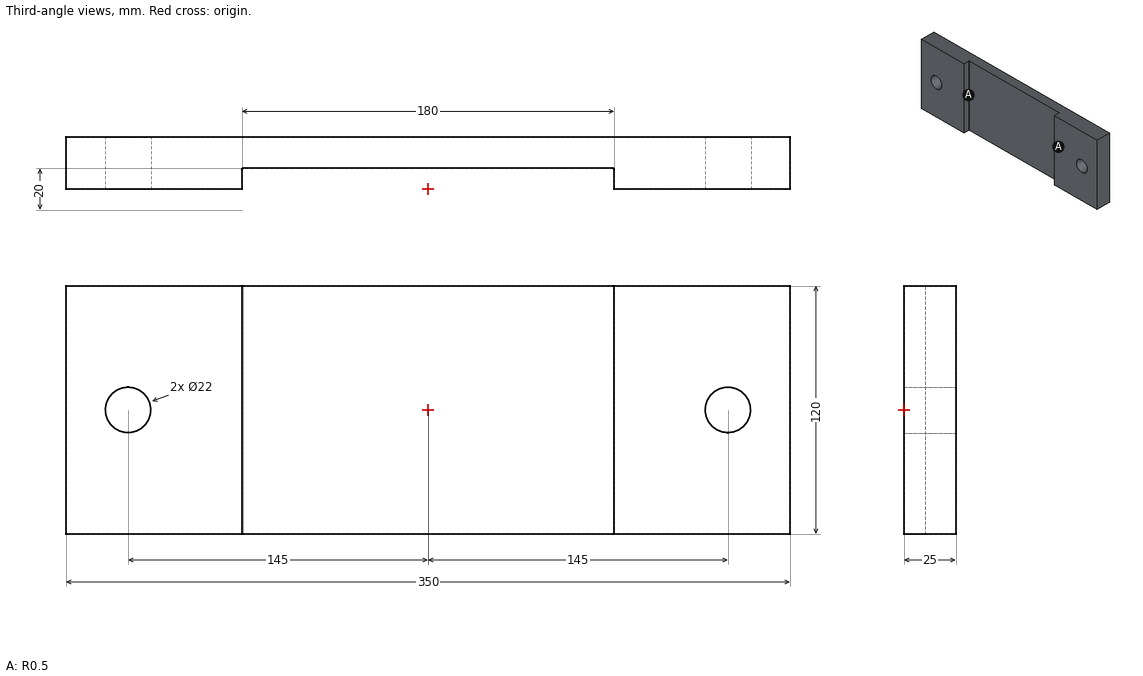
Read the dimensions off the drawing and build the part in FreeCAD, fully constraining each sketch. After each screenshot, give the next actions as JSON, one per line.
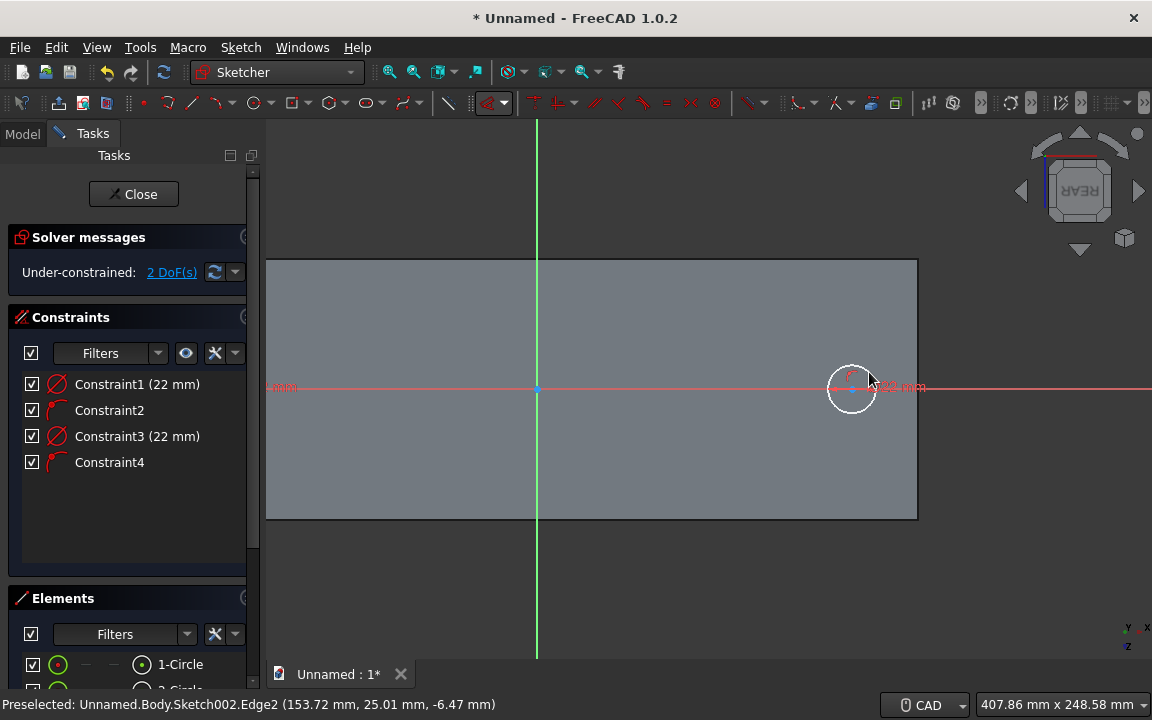
{"action": "left_click", "coordinate": [488, 104]}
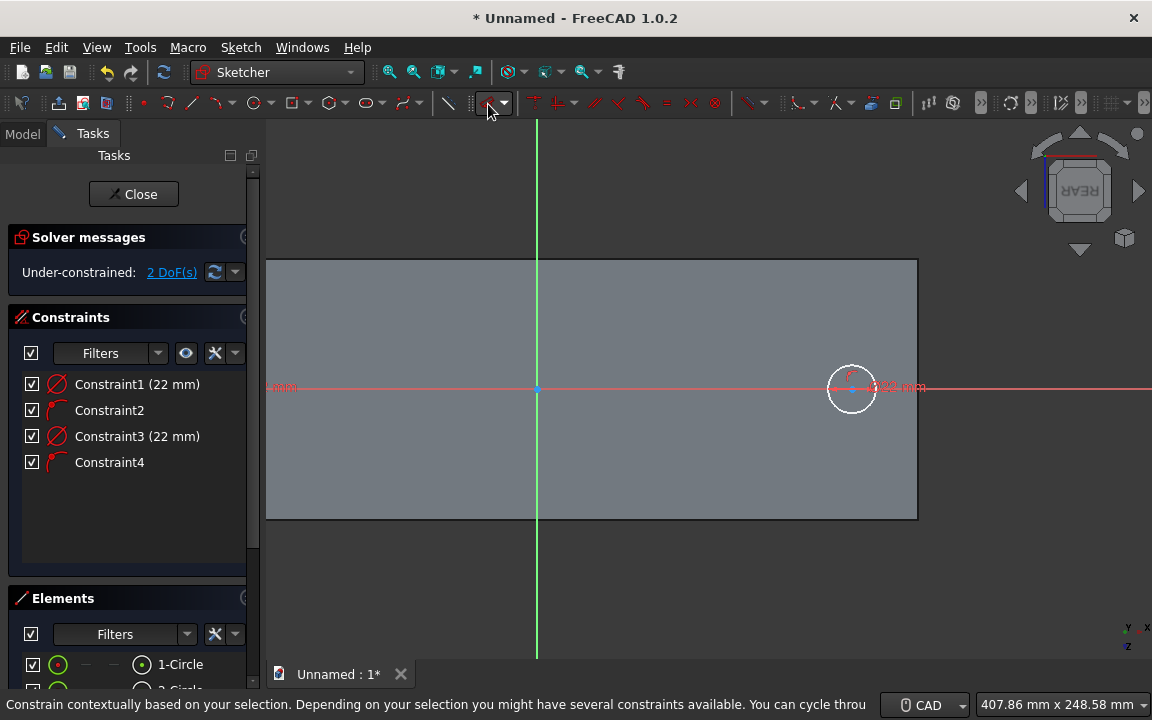
{"action": "scroll", "coordinate": [850, 388], "scroll_direction": "down", "scroll_amount": 2}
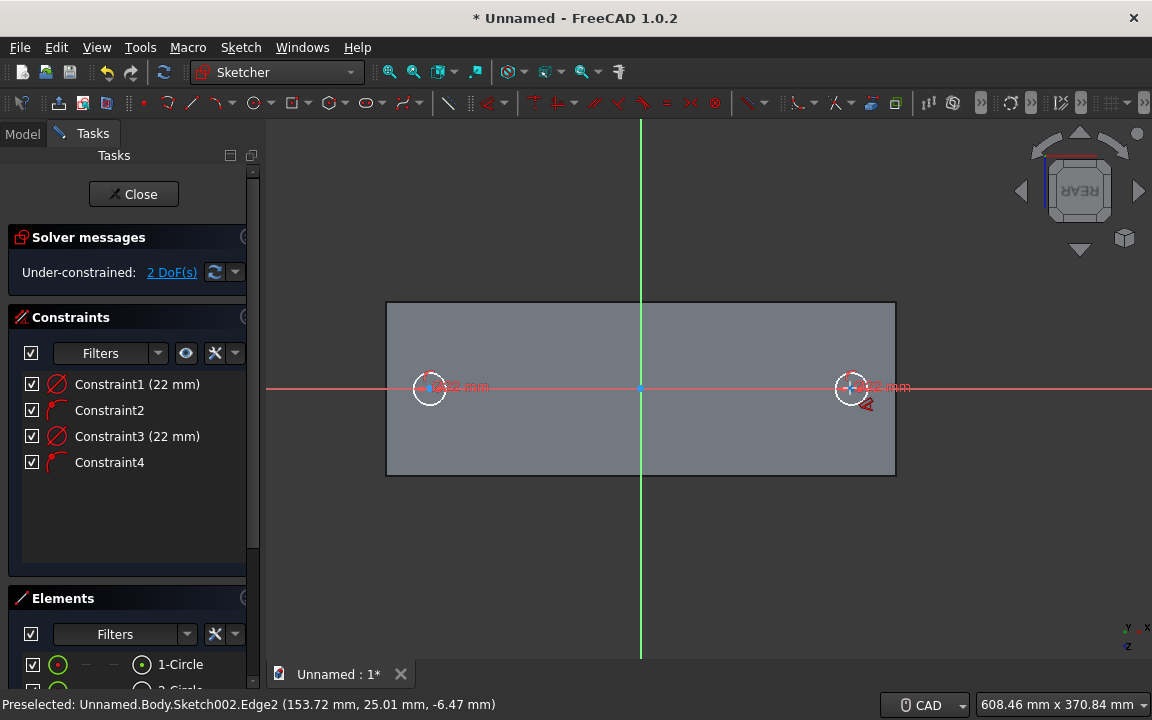
{"action": "left_click", "coordinate": [430, 389]}
{"action": "left_click", "coordinate": [535, 423]}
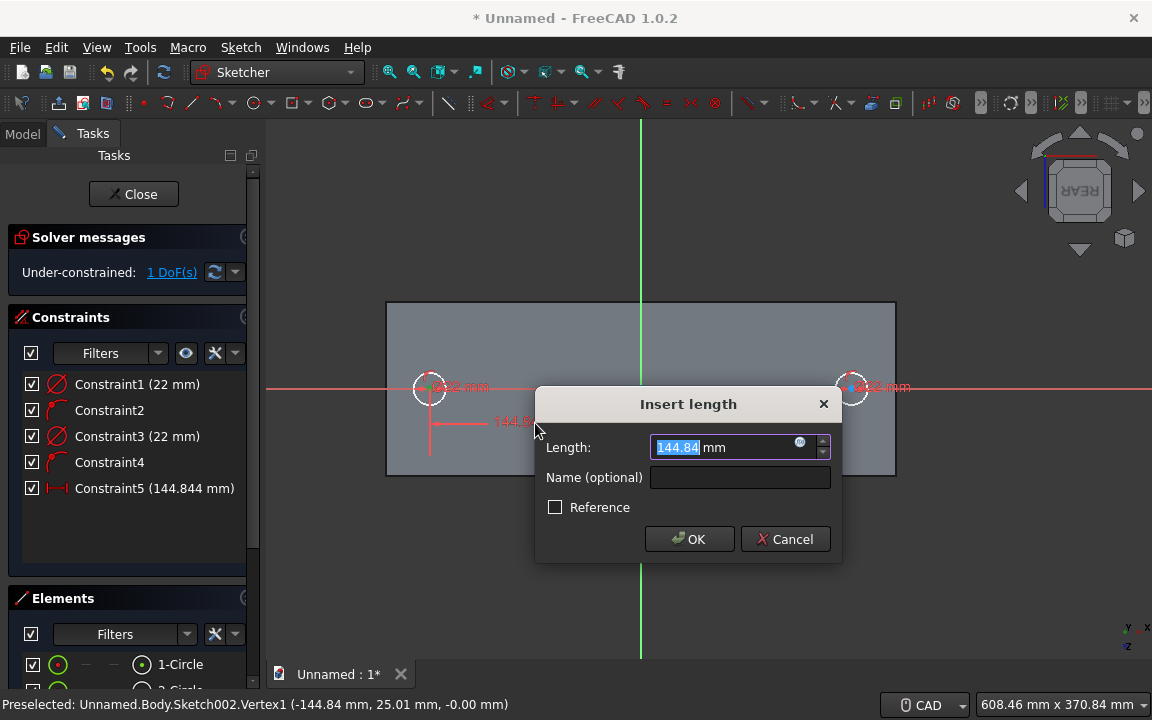
{"action": "type", "text": "145"}
{"action": "key", "text": "Return"}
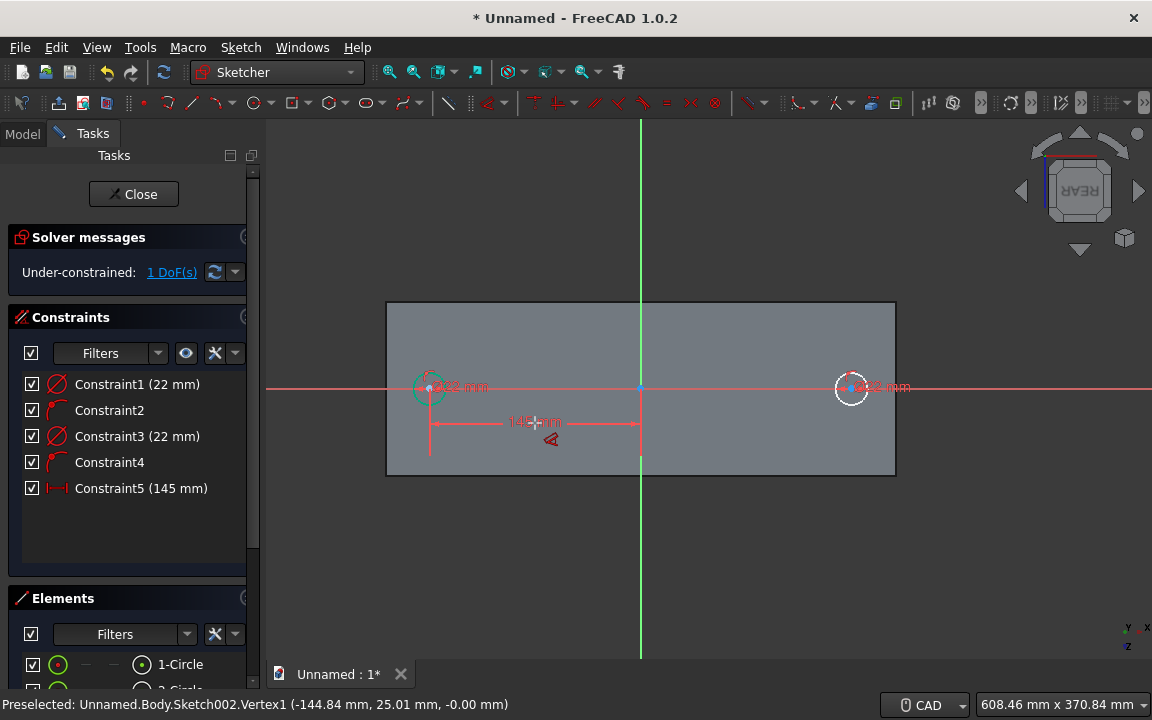
{"action": "left_click", "coordinate": [852, 389]}
{"action": "left_click", "coordinate": [746, 423]}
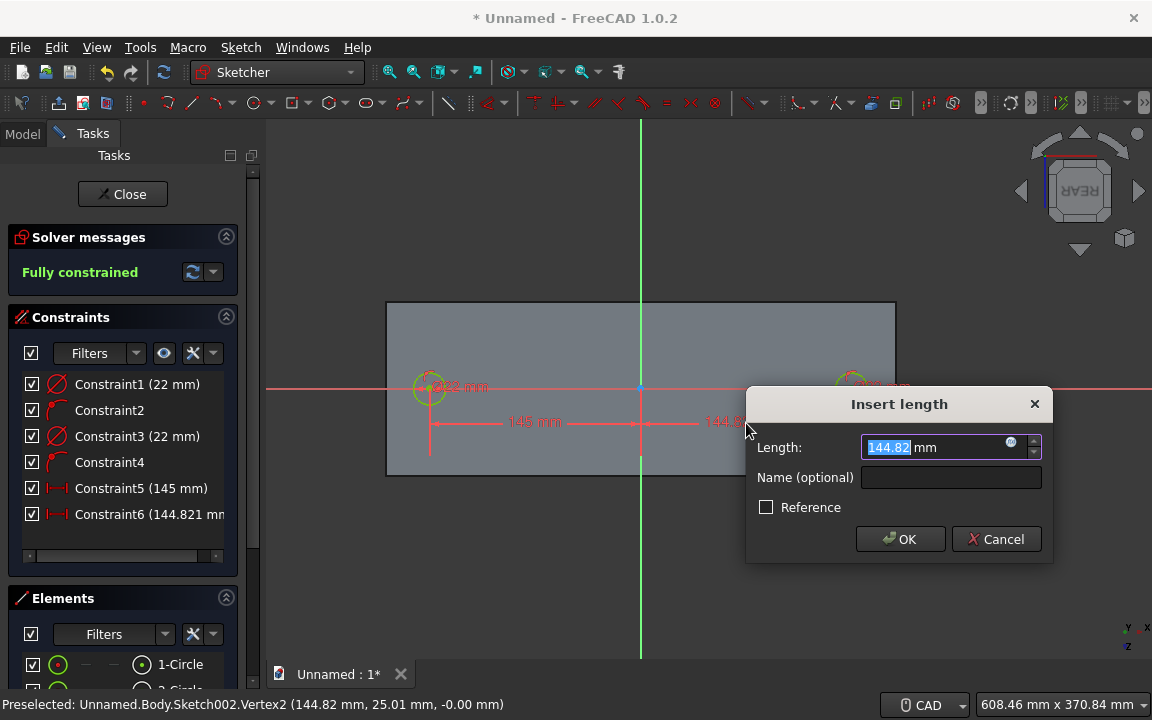
{"action": "type", "text": "145"}
{"action": "key", "text": "Return"}
{"action": "key", "text": "Escape"}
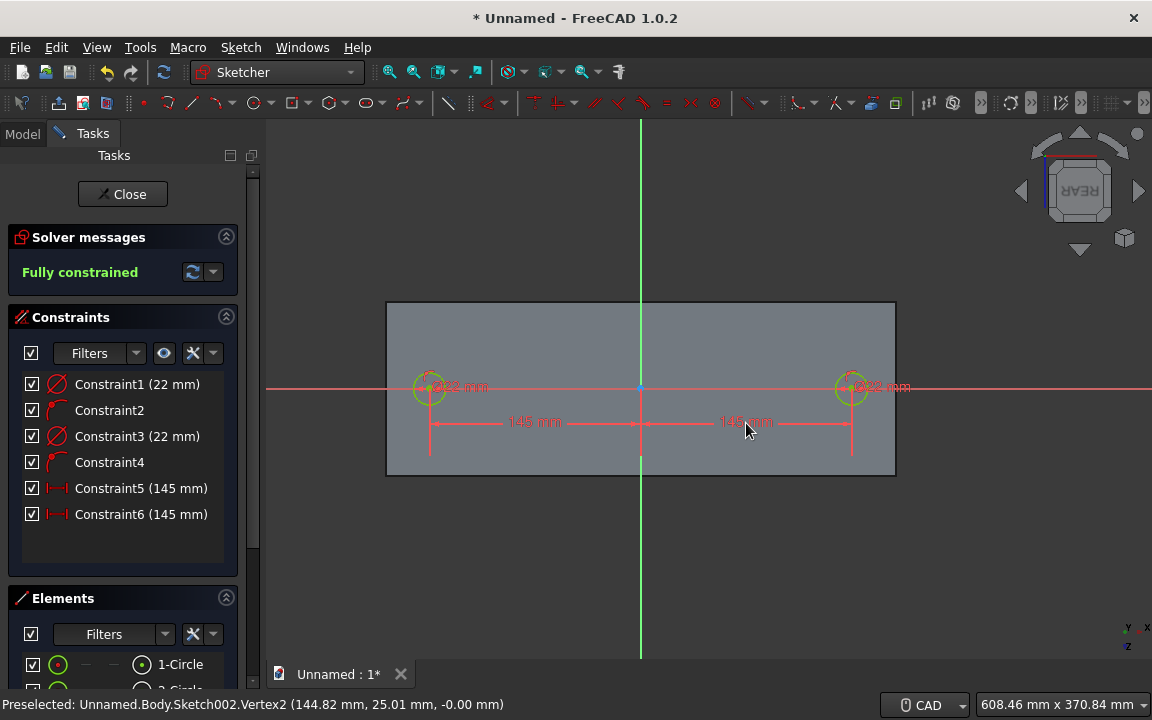
{"action": "left_click", "coordinate": [123, 194]}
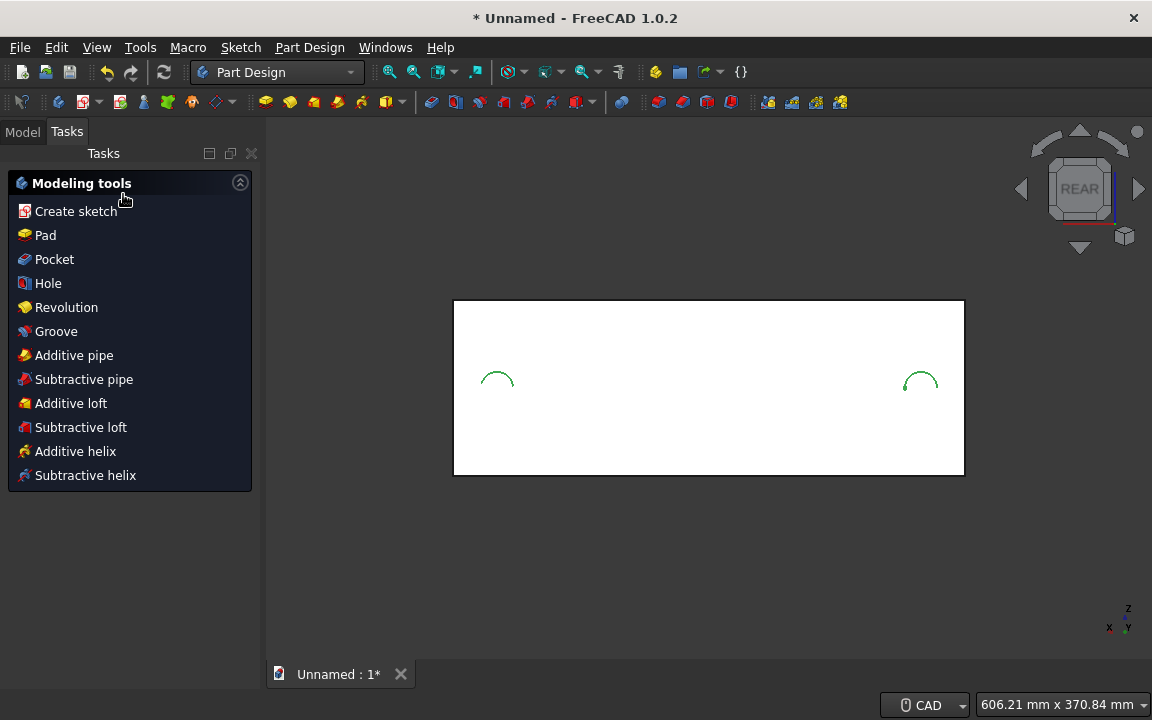
{"action": "left_click", "coordinate": [432, 102]}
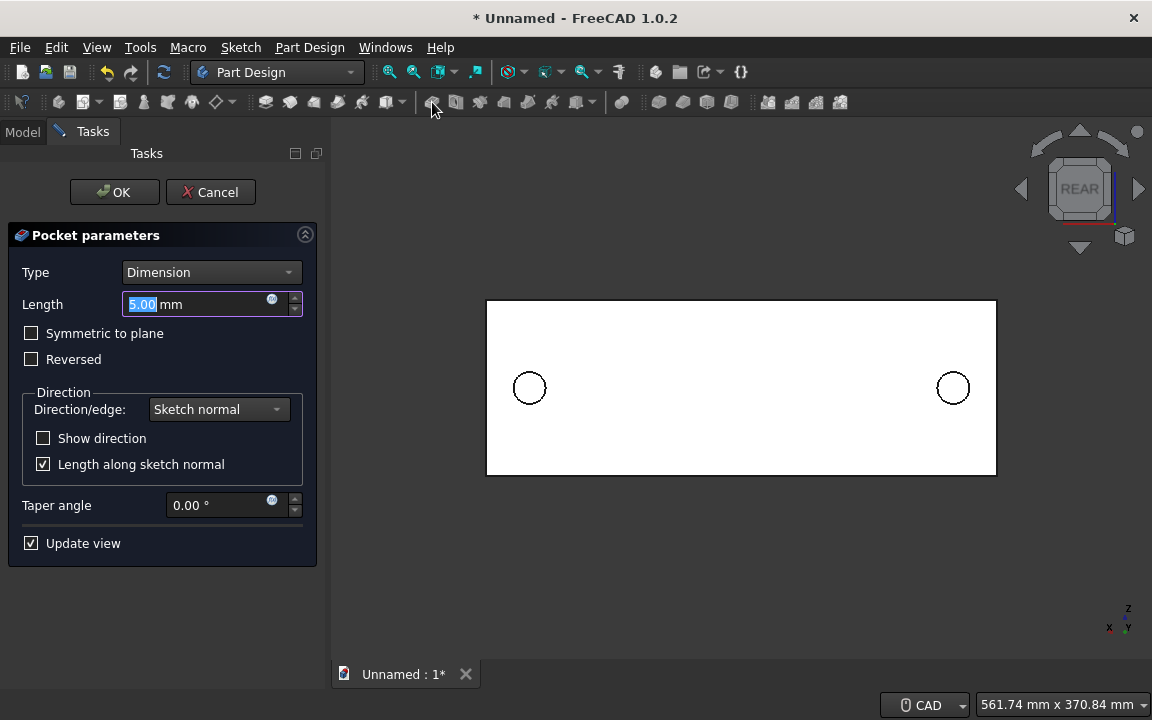
{"action": "type", "text": "25"}
{"action": "key", "text": "Tab"}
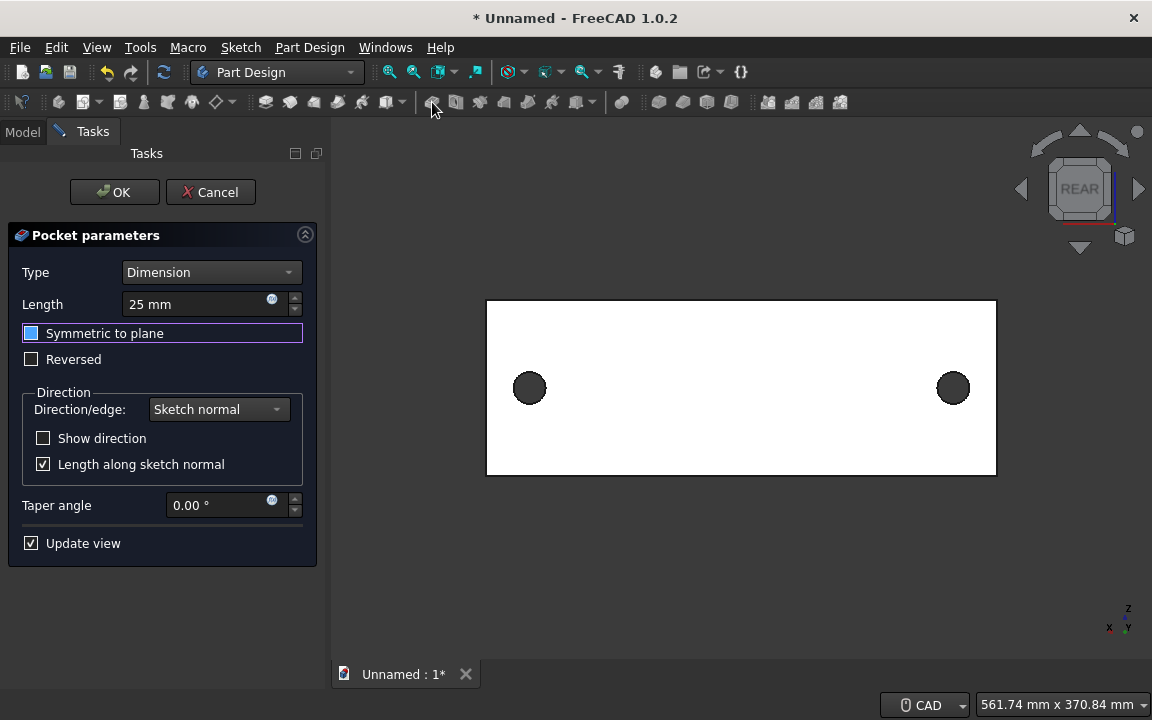
{"action": "left_click", "coordinate": [115, 192]}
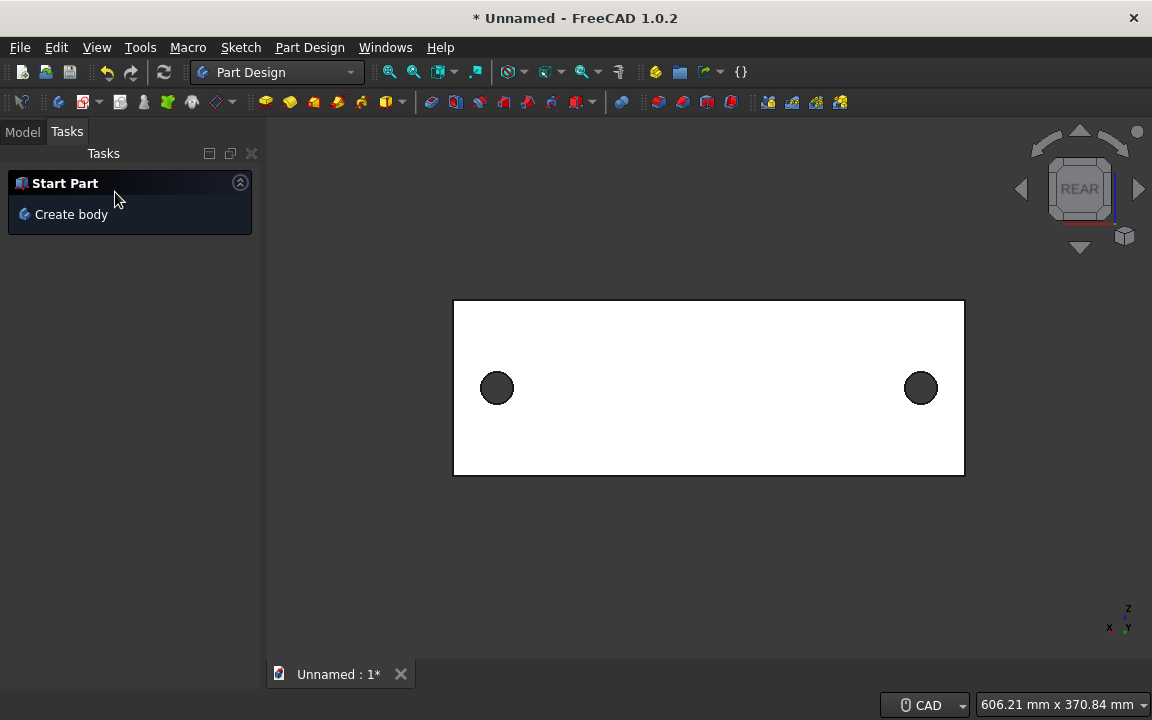
{"action": "key", "text": "0"}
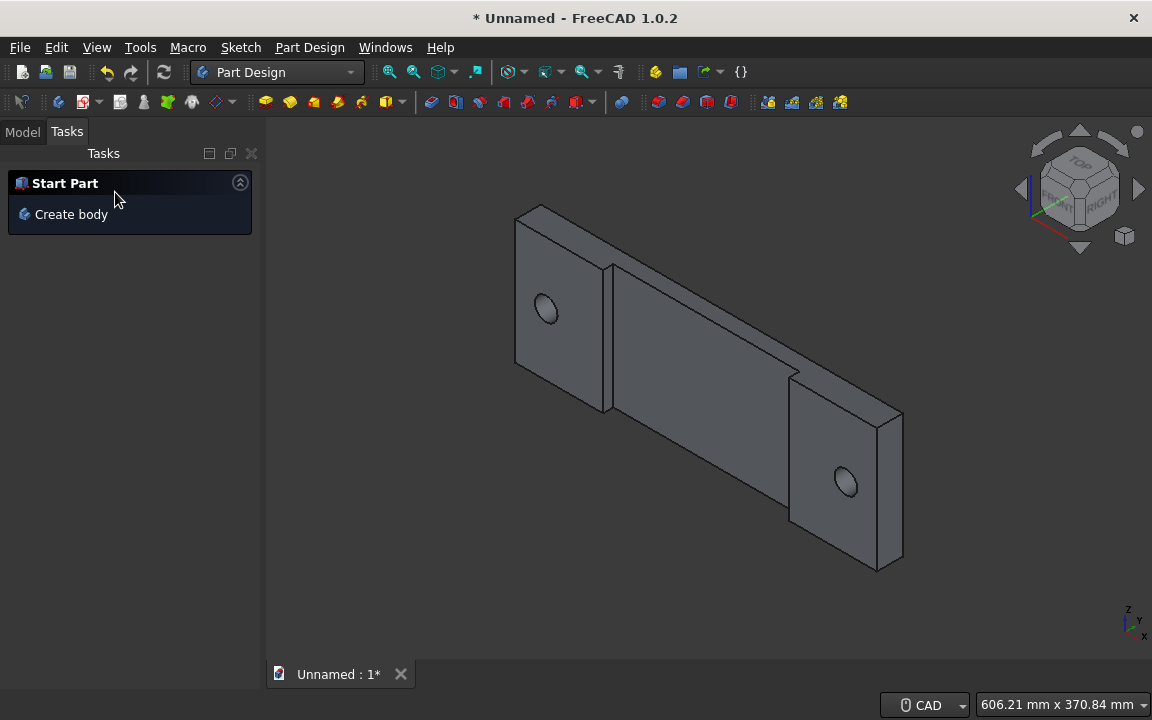
{"action": "key", "text": "2"}